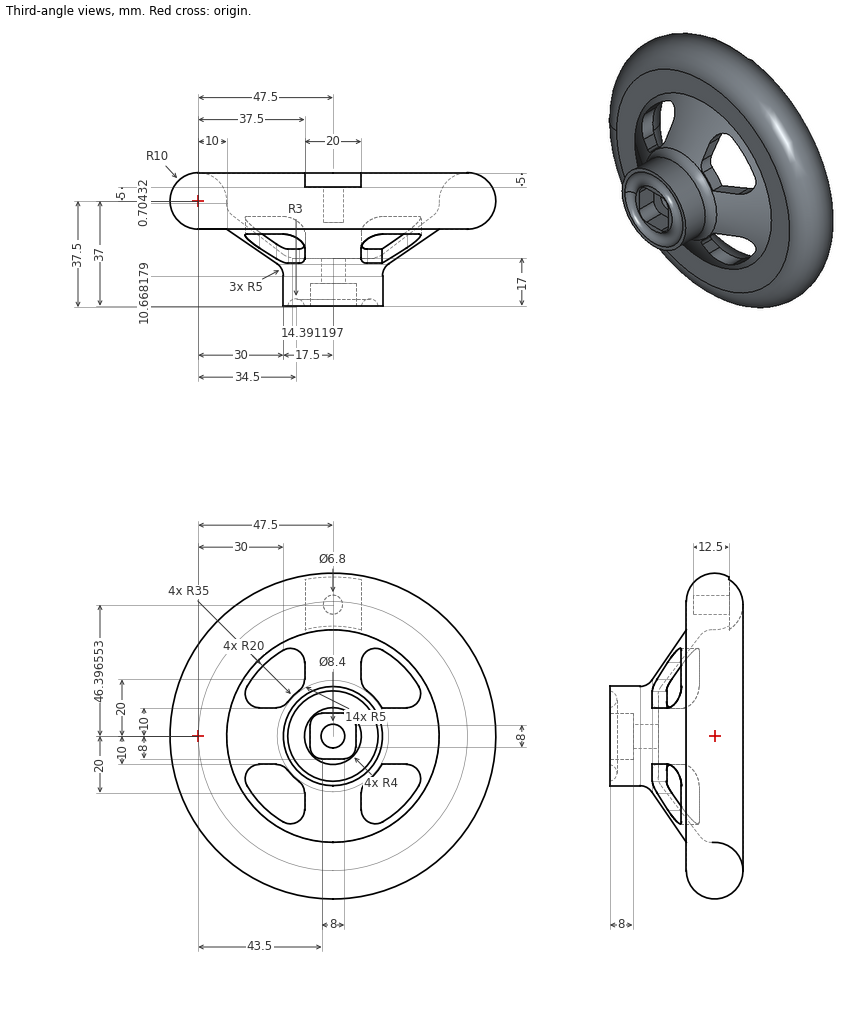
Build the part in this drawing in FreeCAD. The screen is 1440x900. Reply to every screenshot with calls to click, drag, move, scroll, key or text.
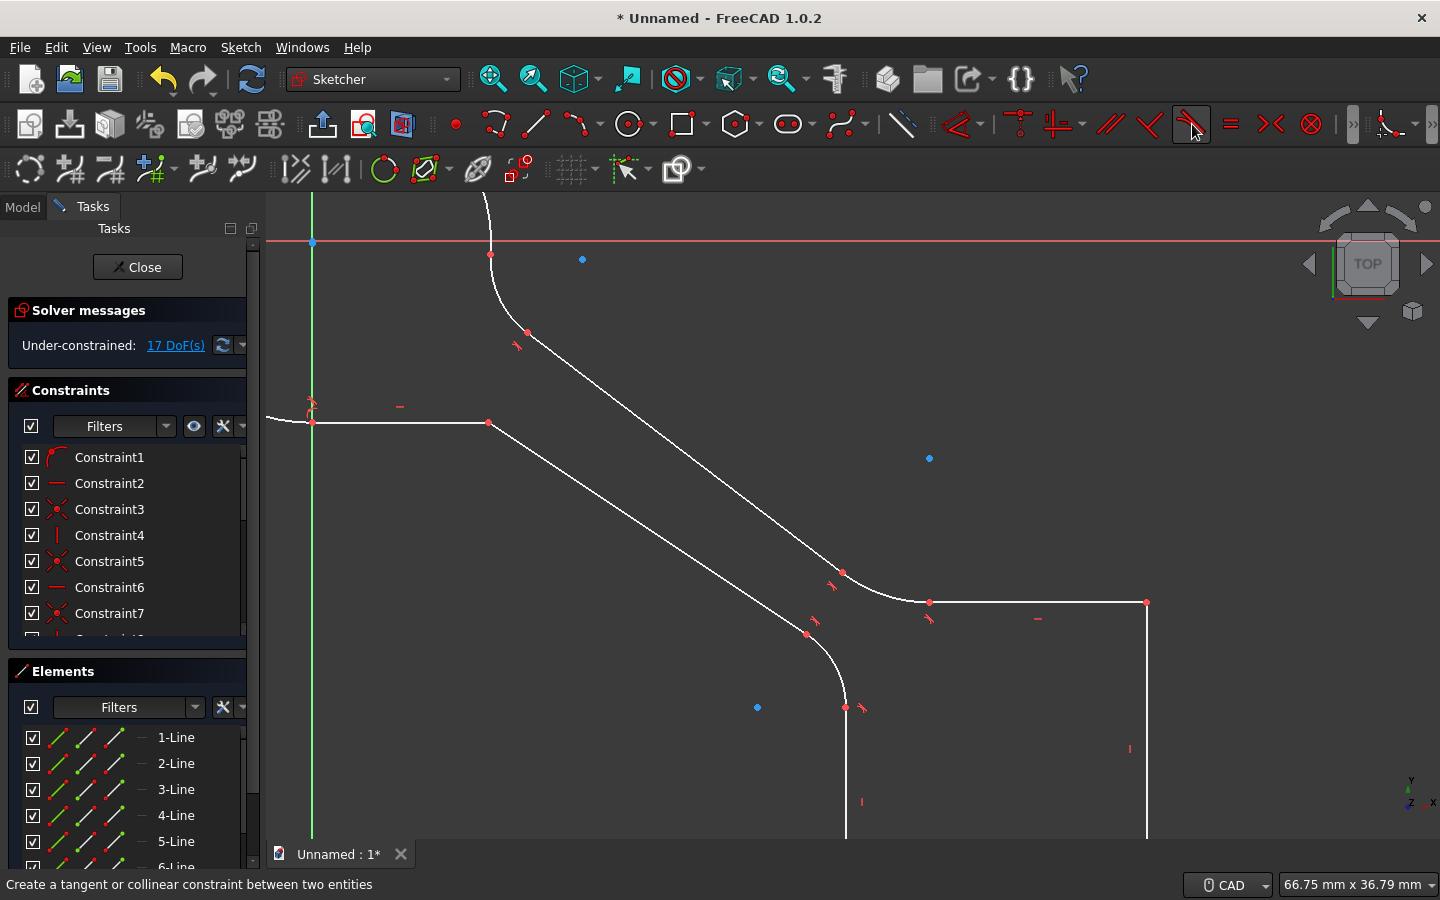
click(493, 281)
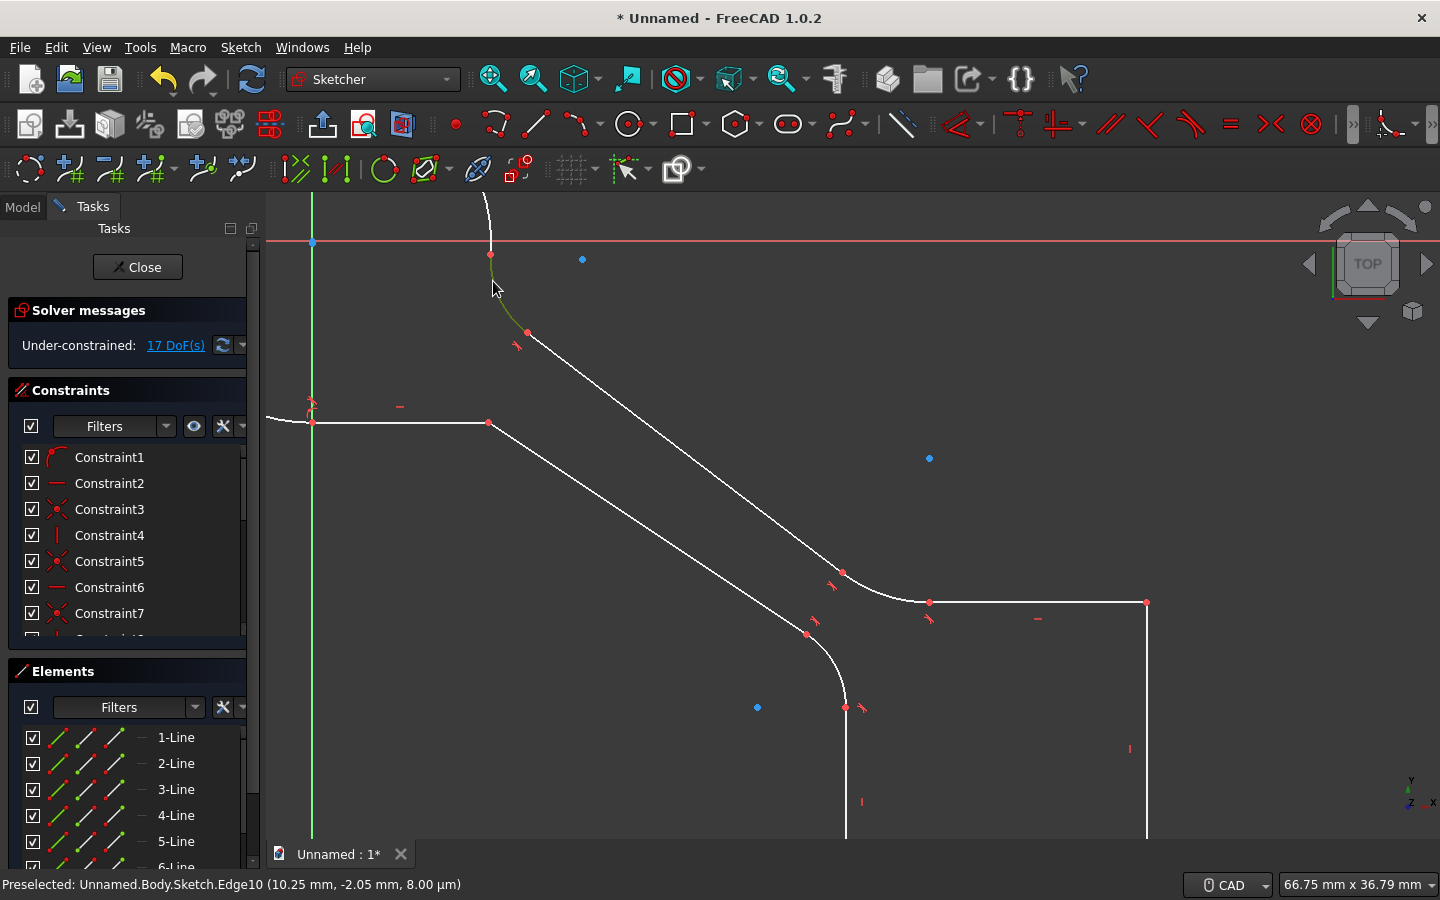
scroll(851, 614, down, 5)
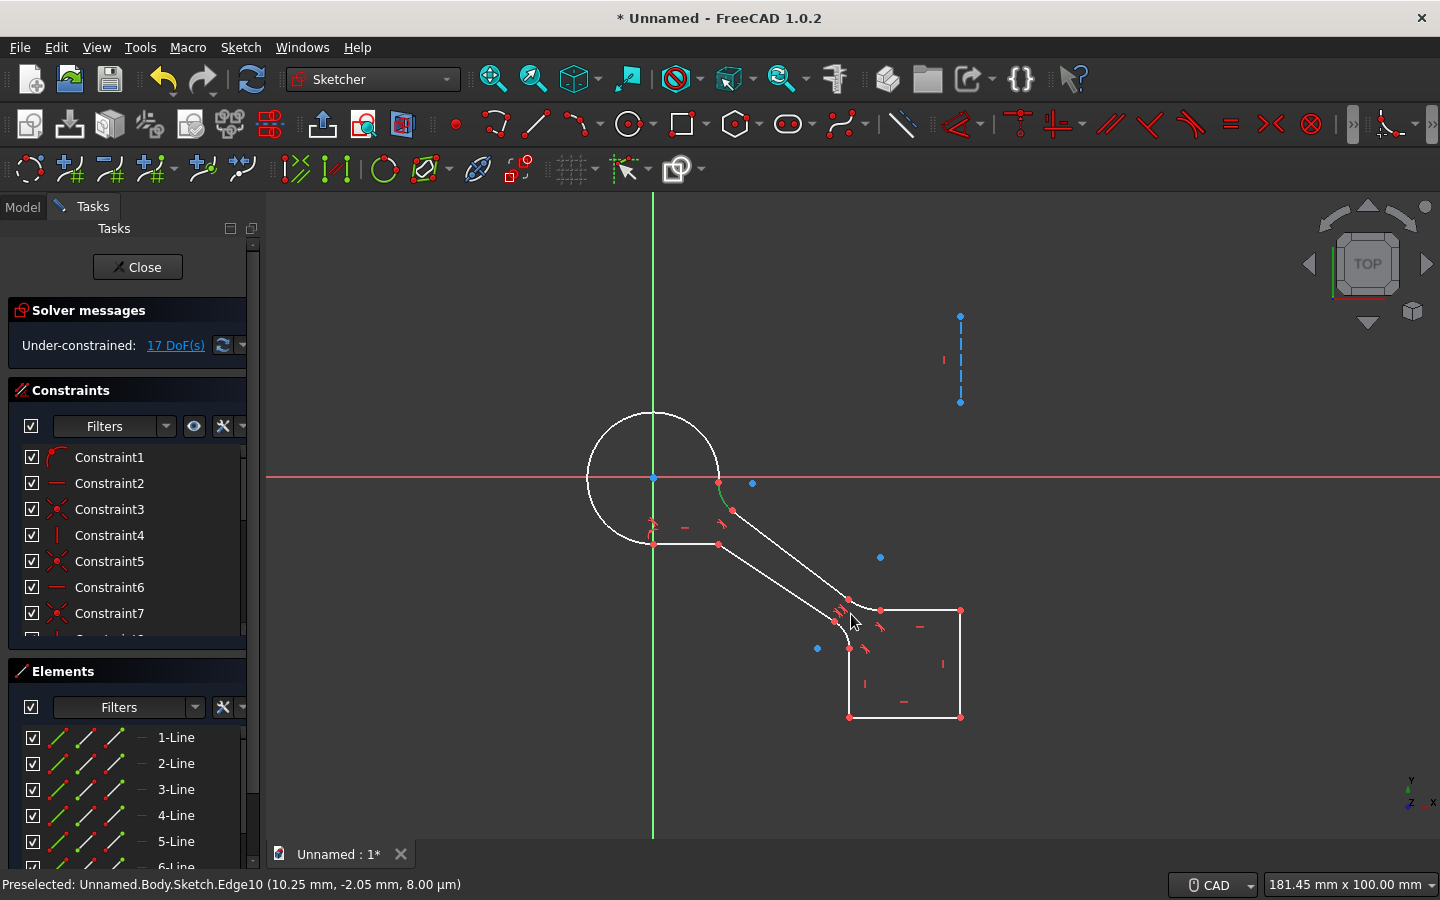
click(666, 414)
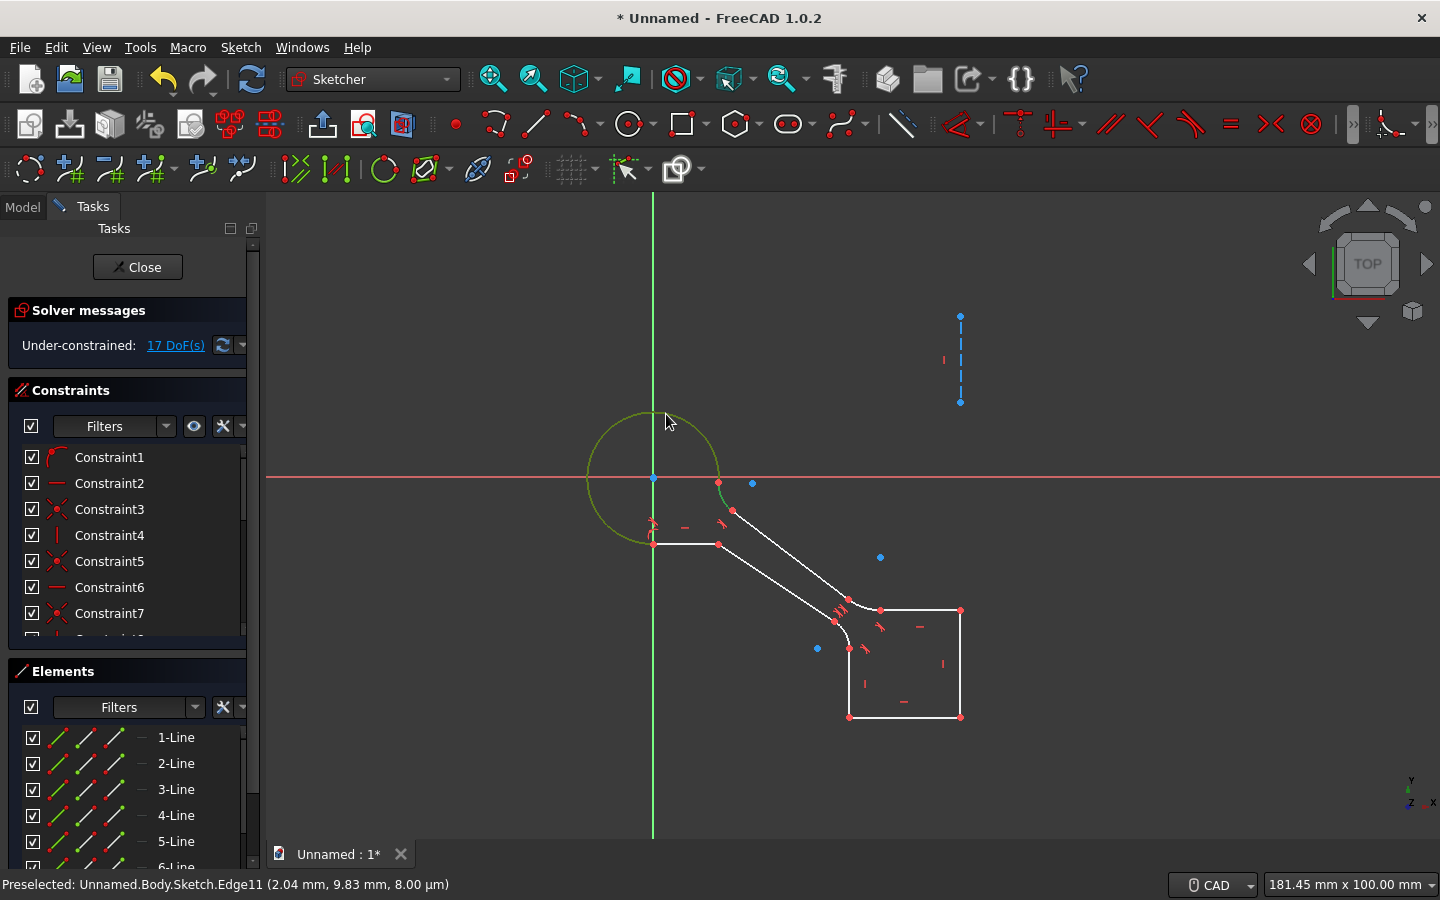
click(1192, 124)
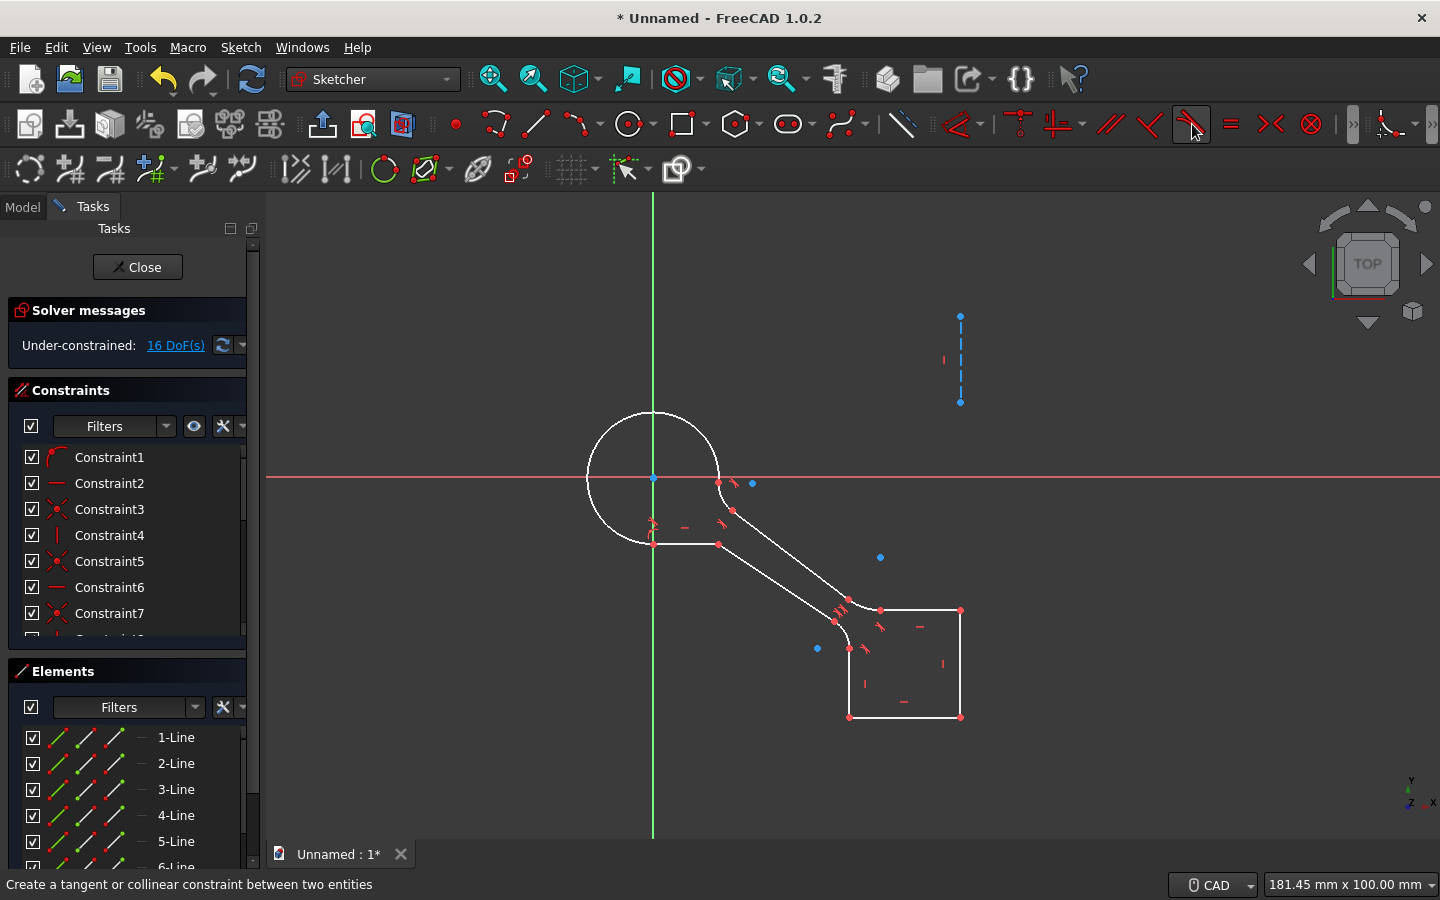
scroll(848, 639, up, 2)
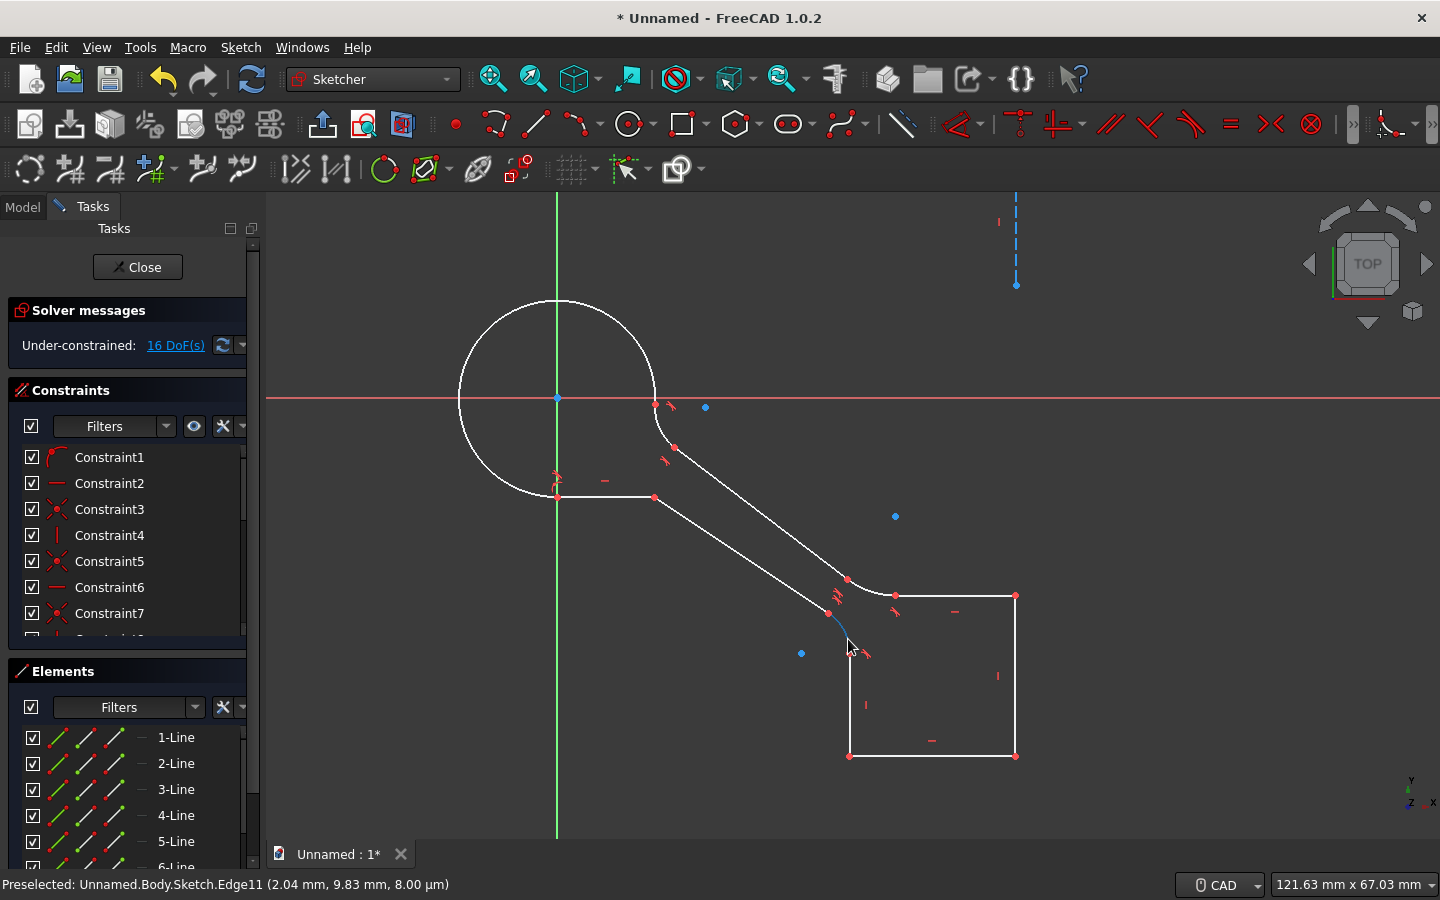
click(848, 639)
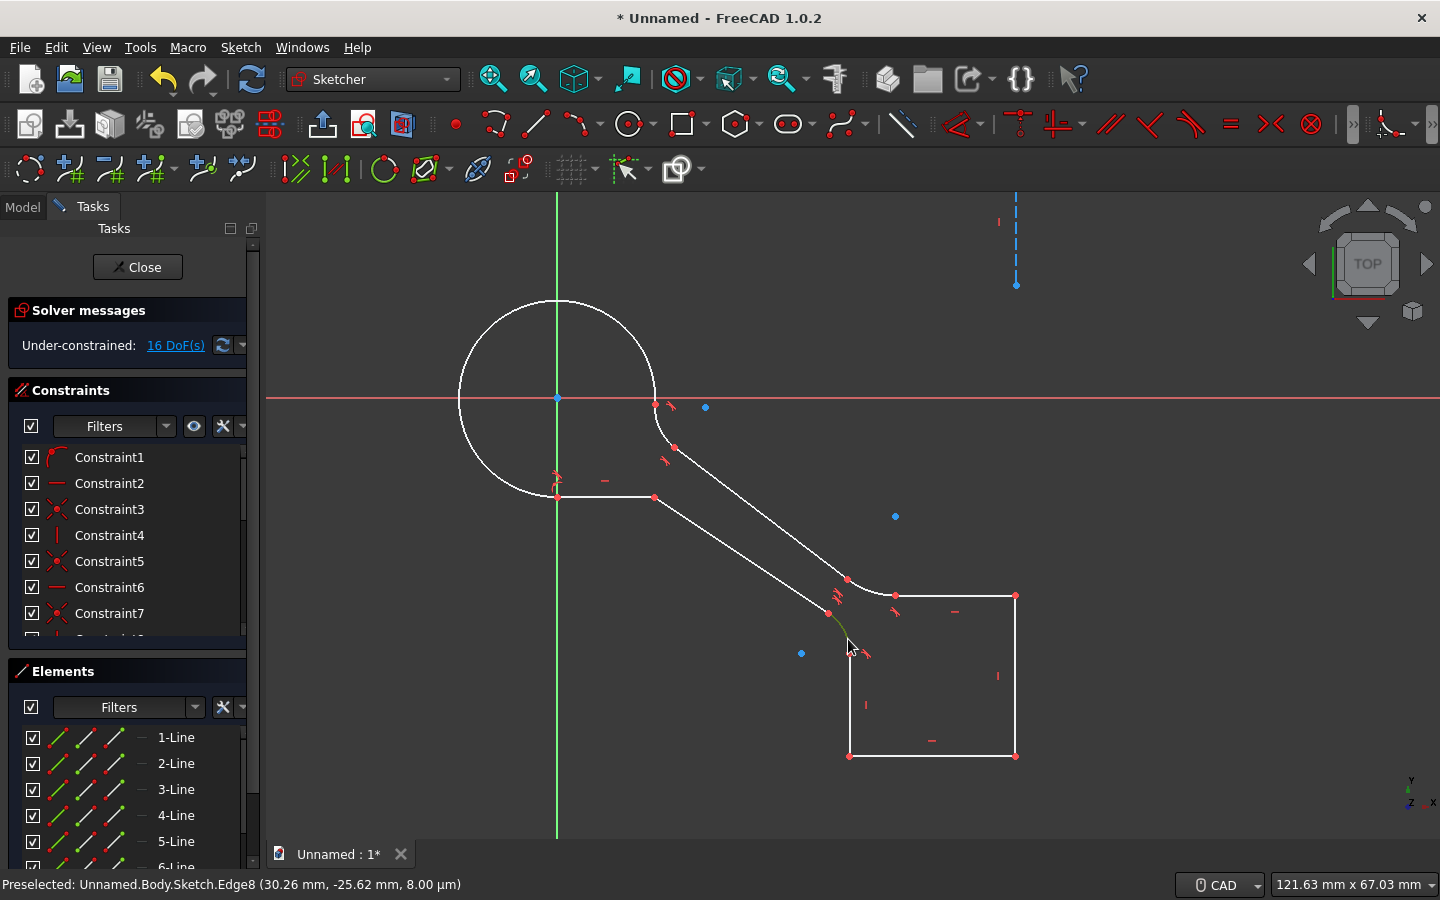
click(861, 588)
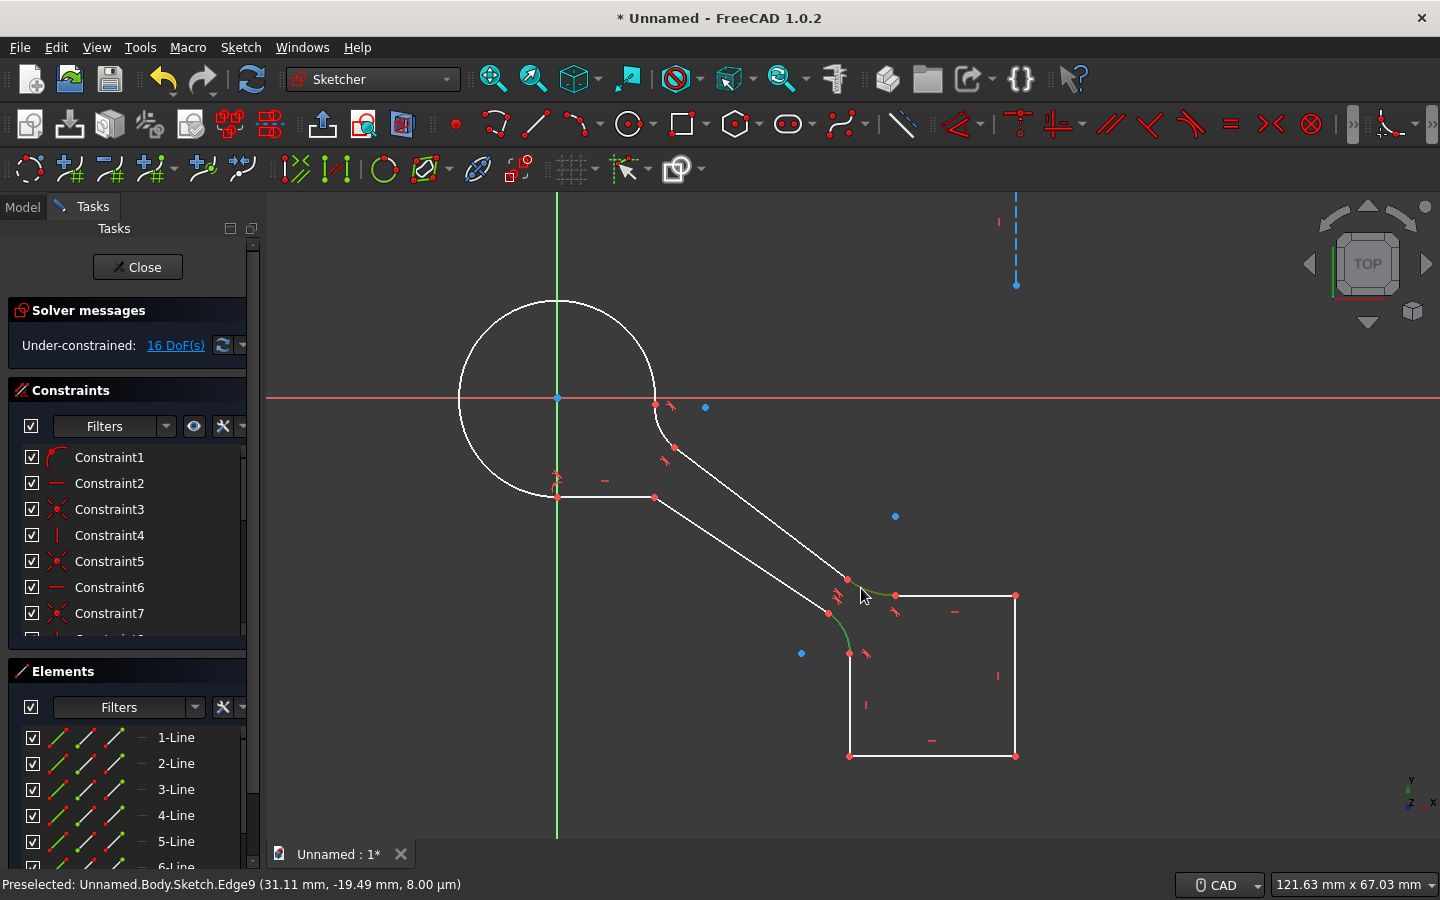
click(656, 419)